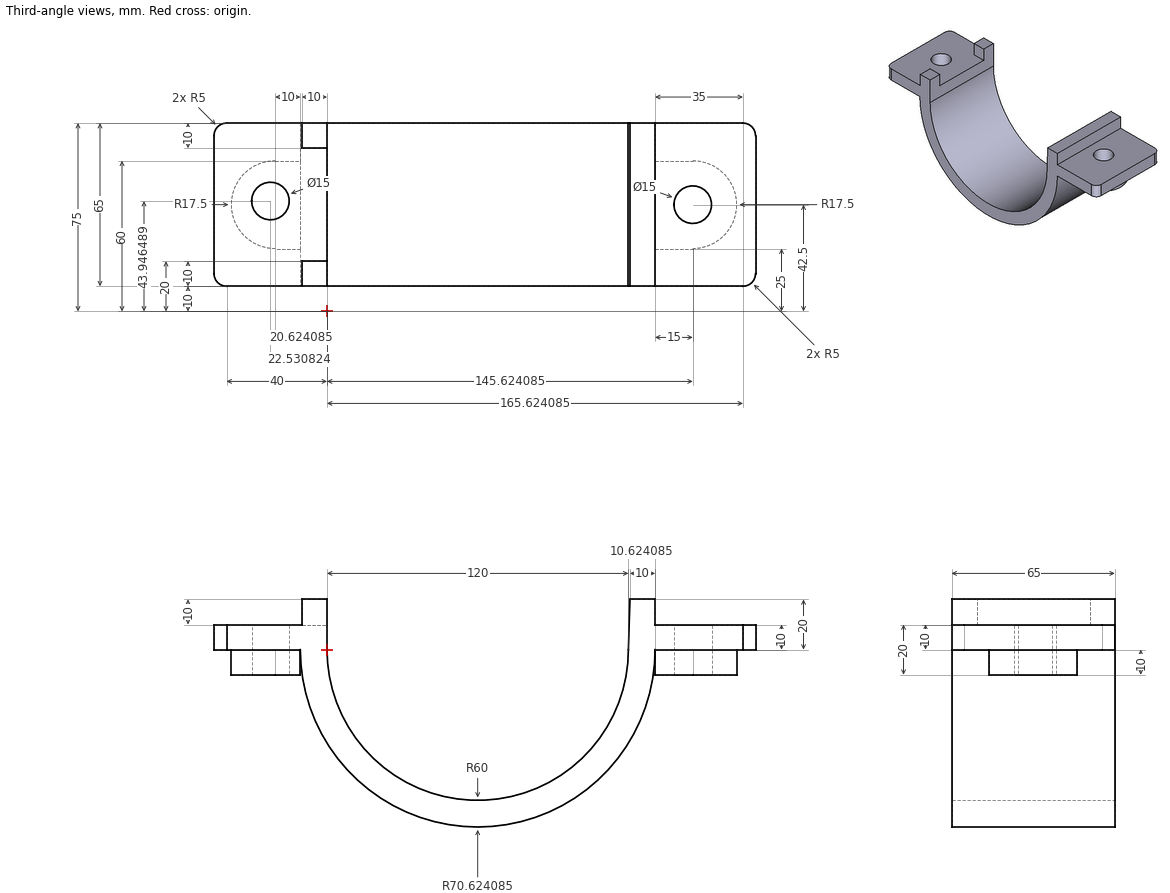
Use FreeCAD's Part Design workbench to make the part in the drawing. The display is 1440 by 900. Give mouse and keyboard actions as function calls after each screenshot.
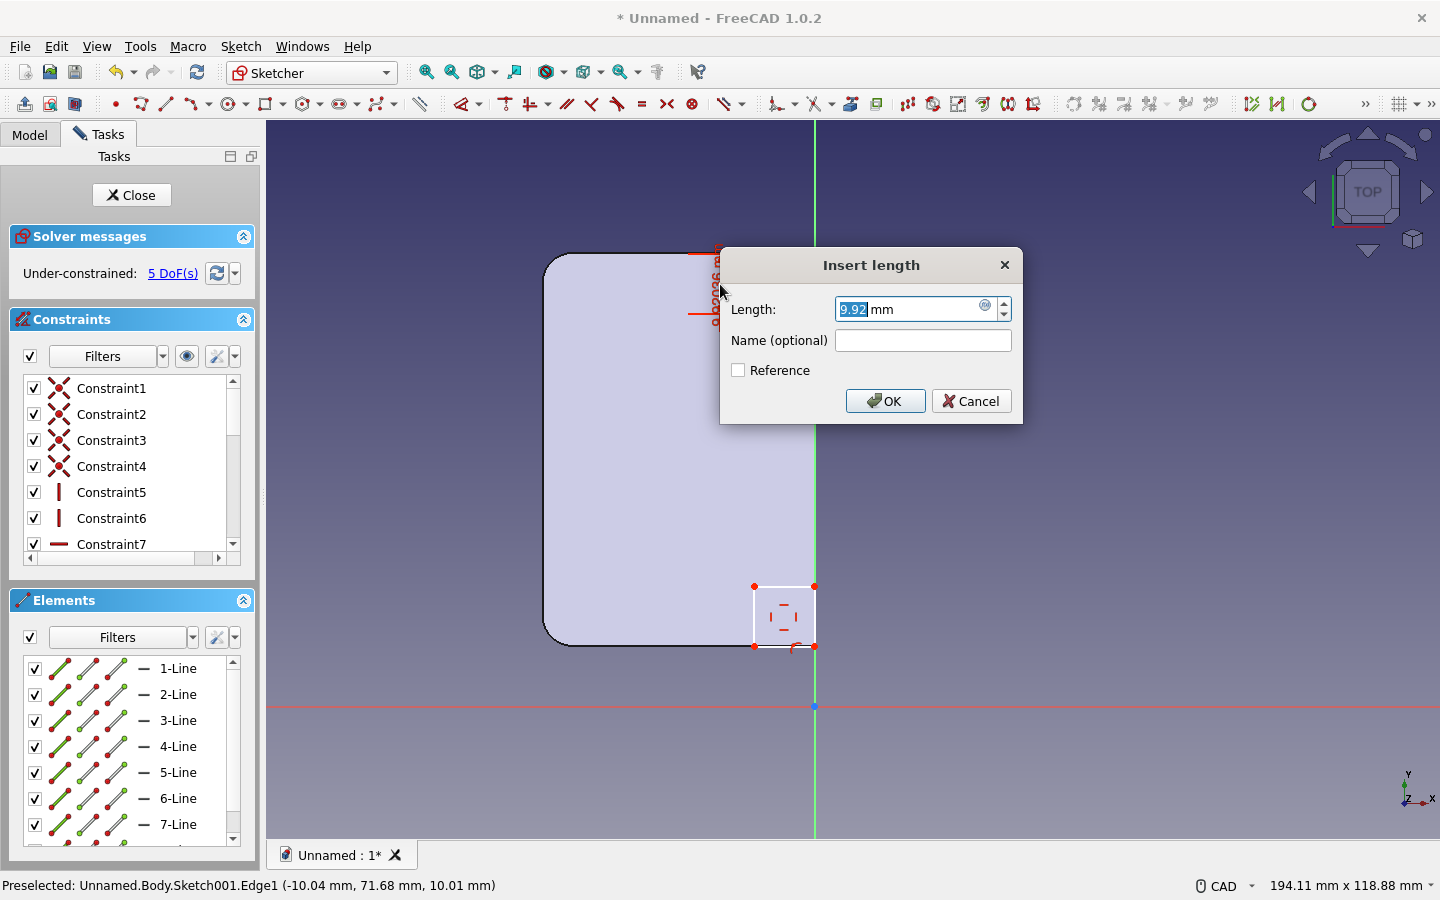
text(10)
key(Return)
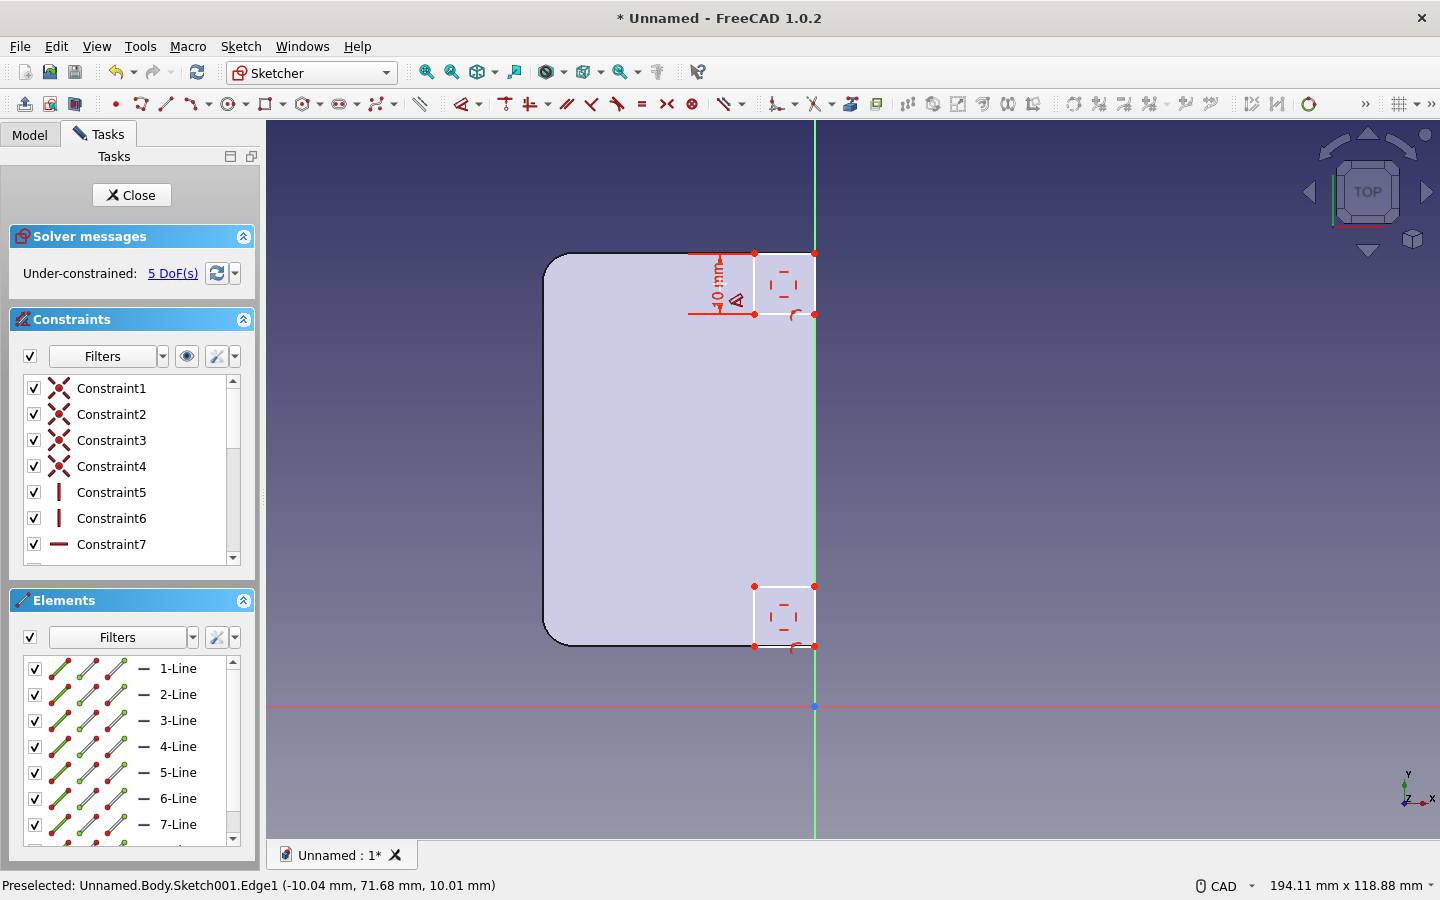
click(772, 314)
click(798, 280)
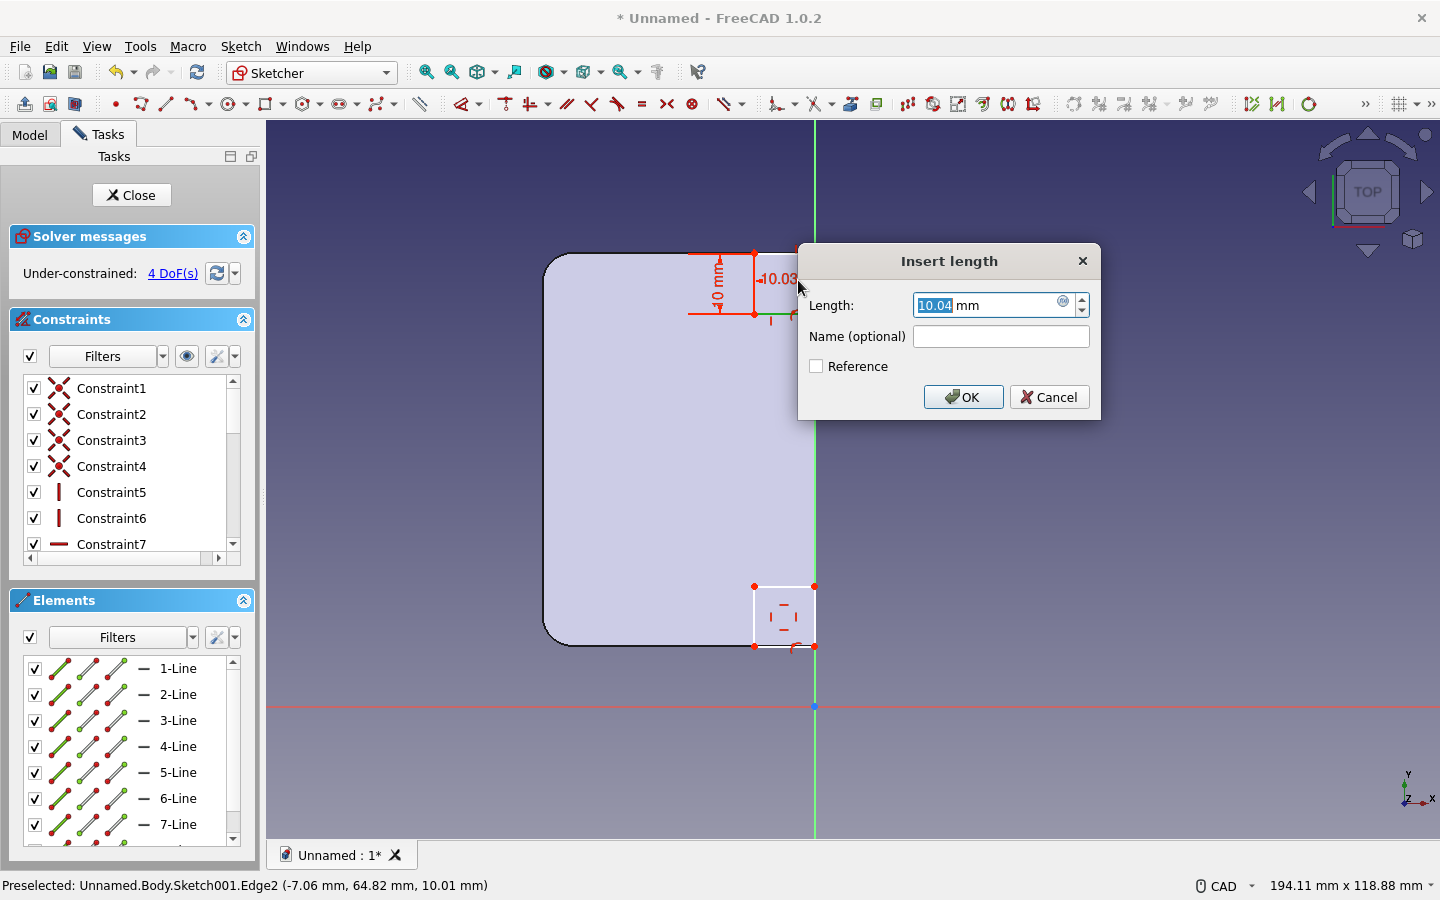
text(10)
key(Return)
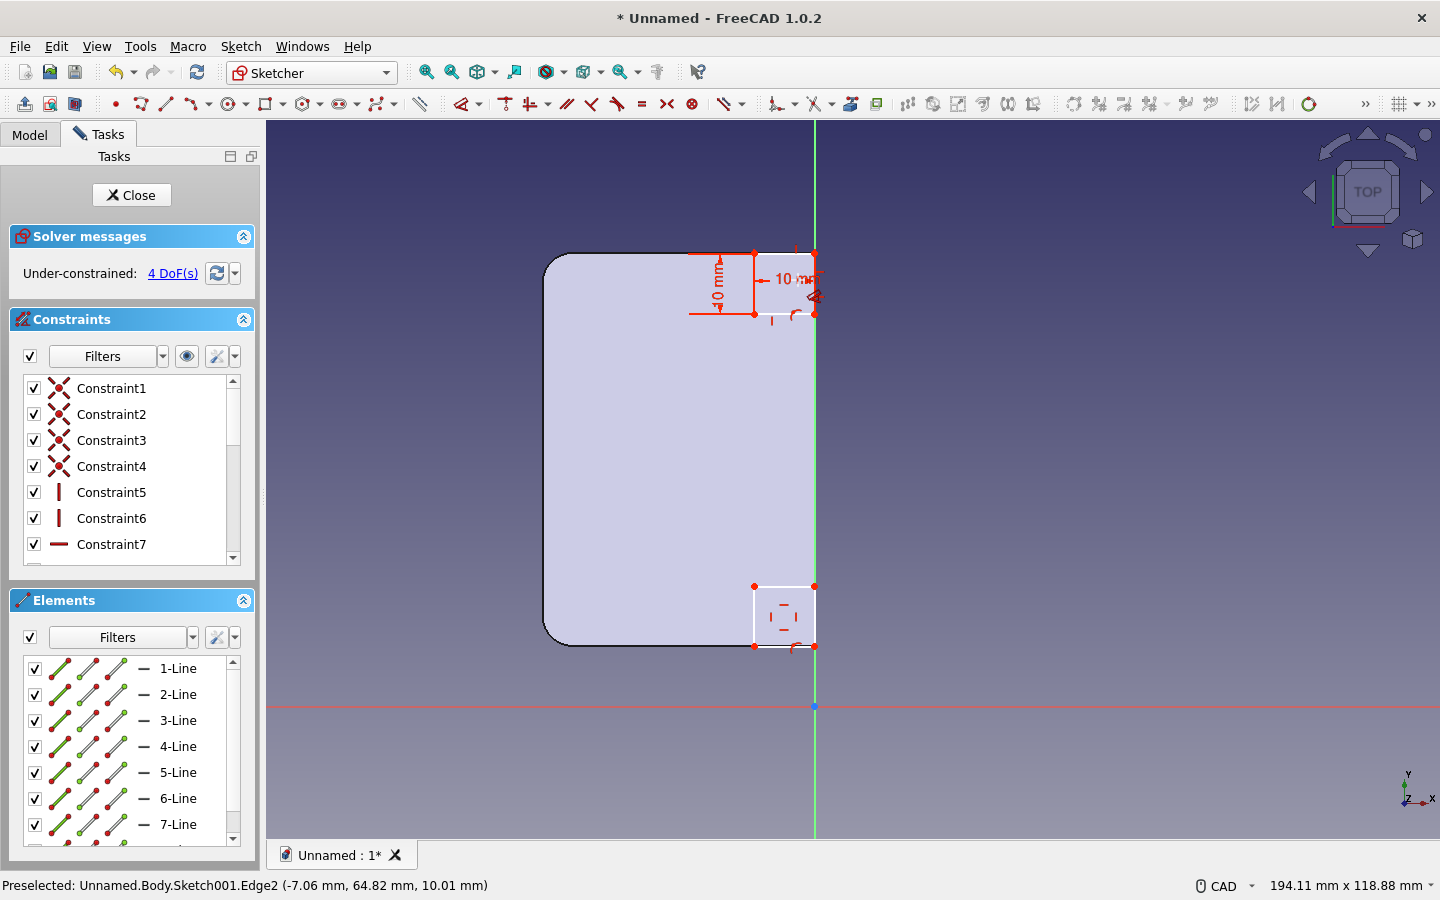
click(754, 605)
click(720, 617)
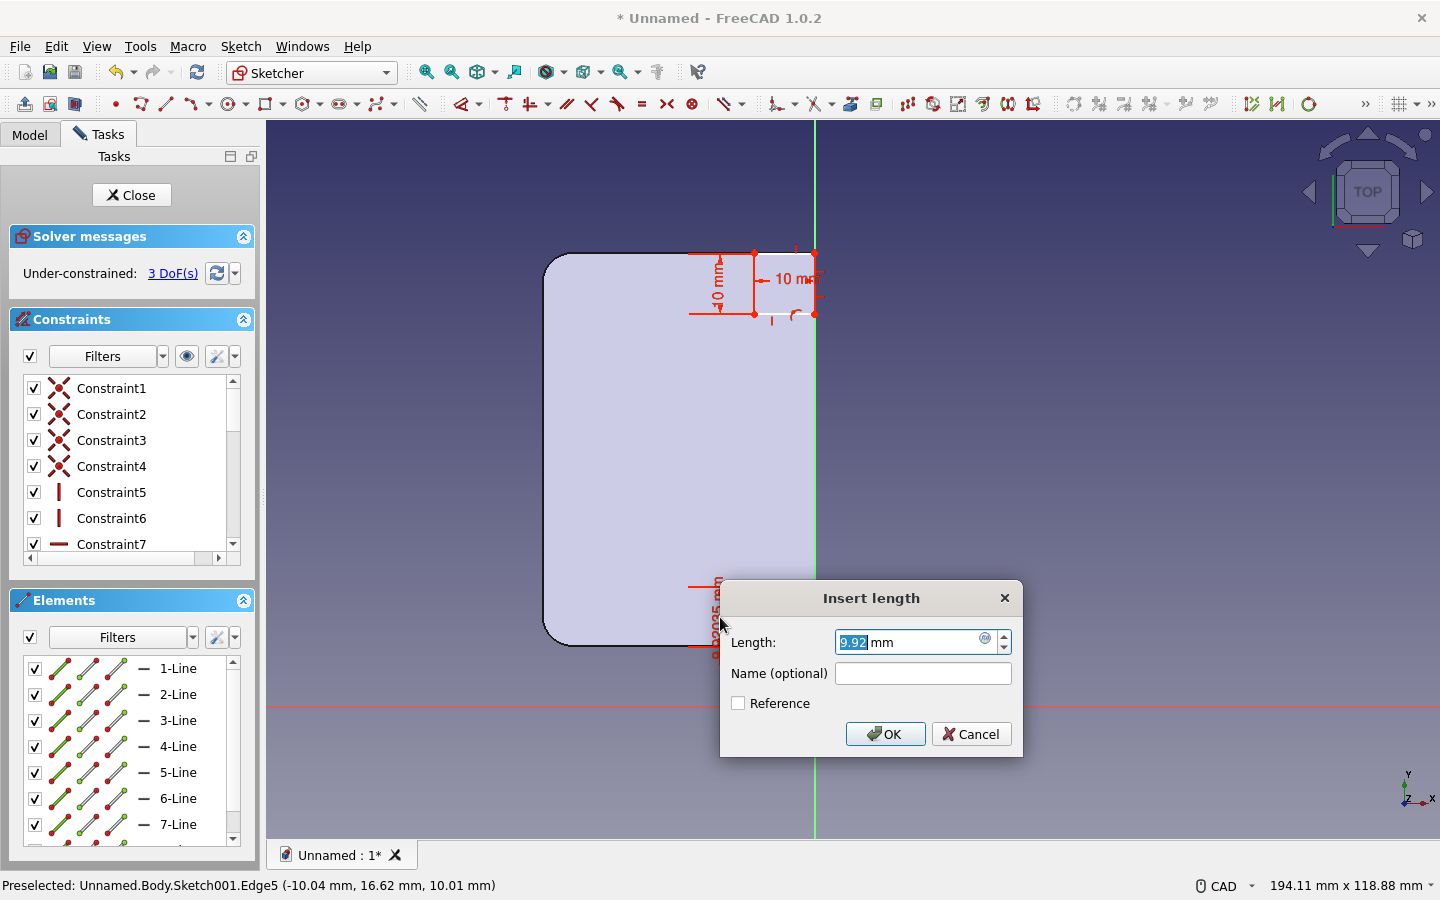
text(10)
key(Return)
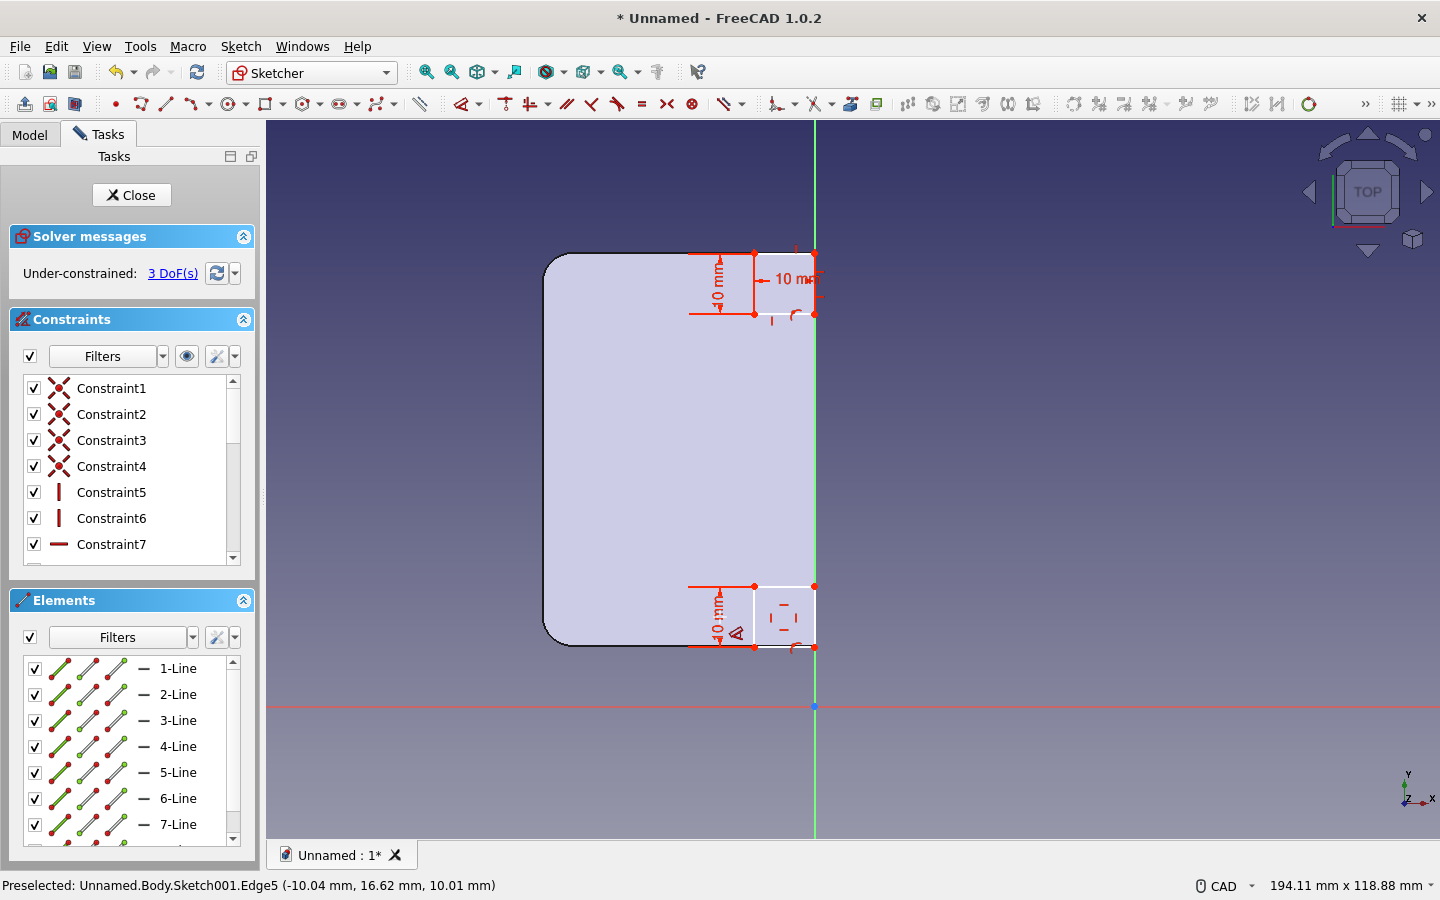
click(772, 647)
click(784, 681)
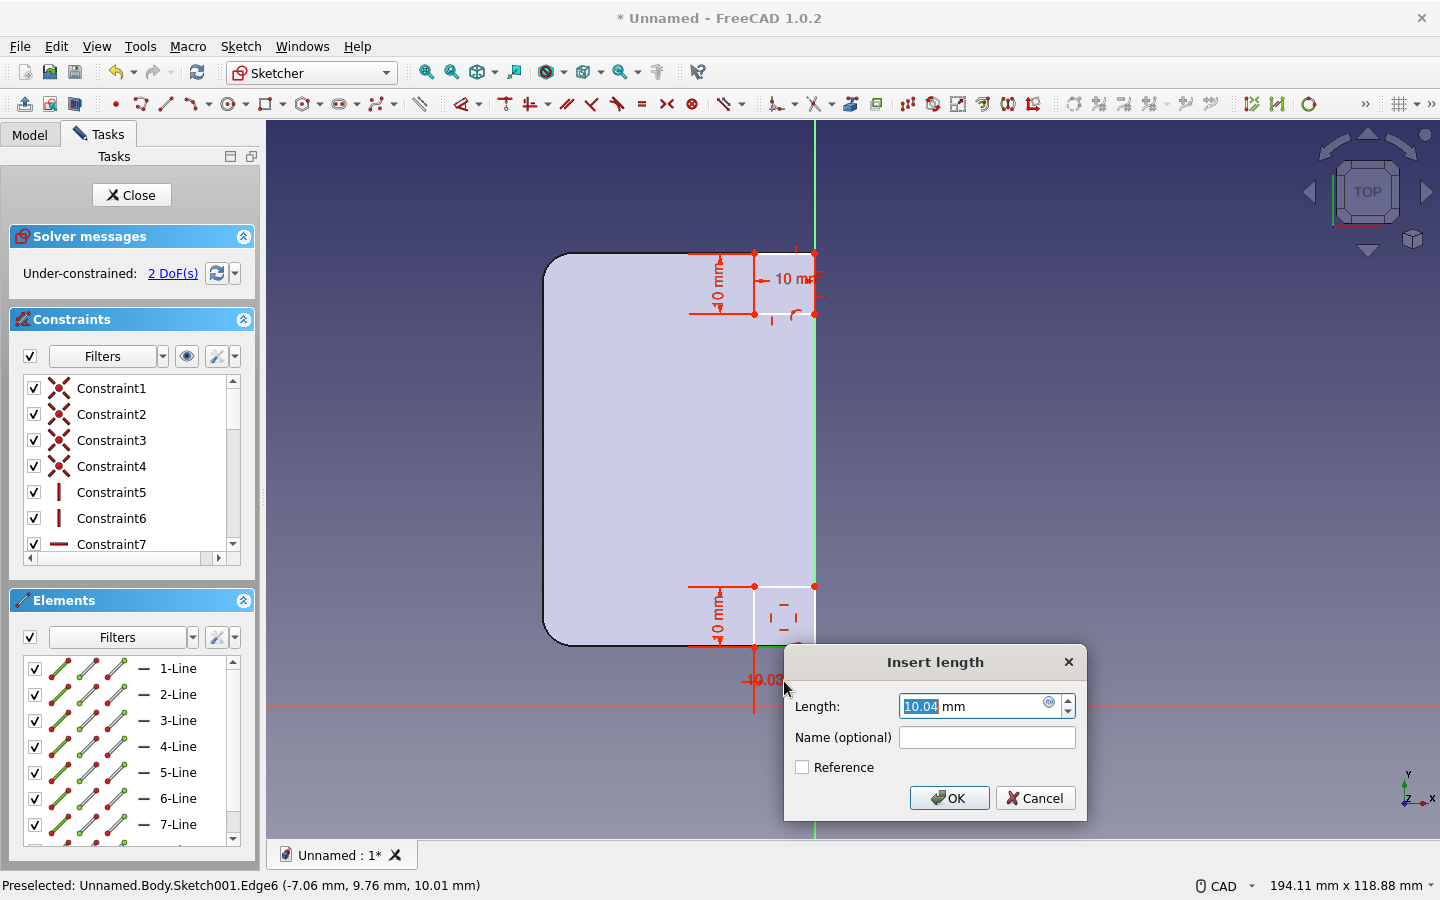
text(10)
key(Return)